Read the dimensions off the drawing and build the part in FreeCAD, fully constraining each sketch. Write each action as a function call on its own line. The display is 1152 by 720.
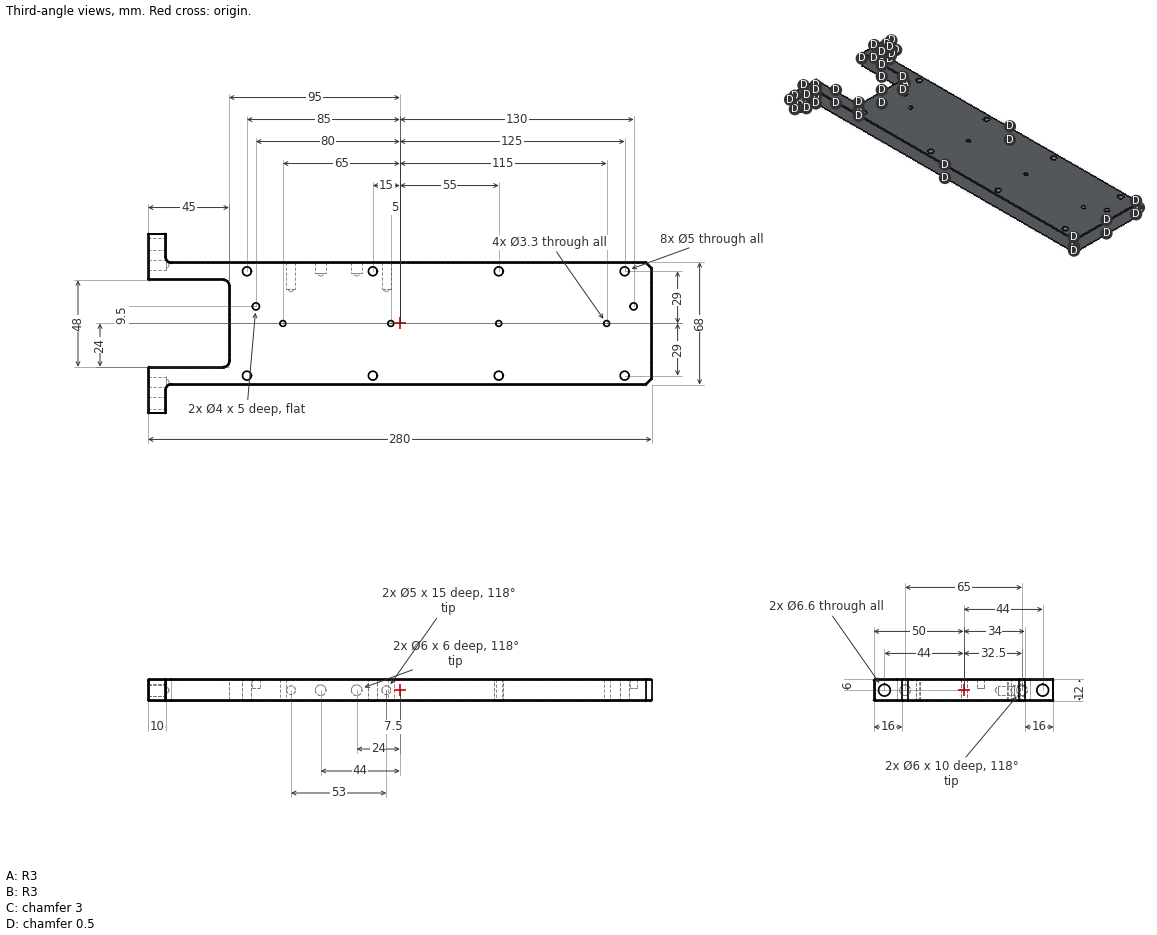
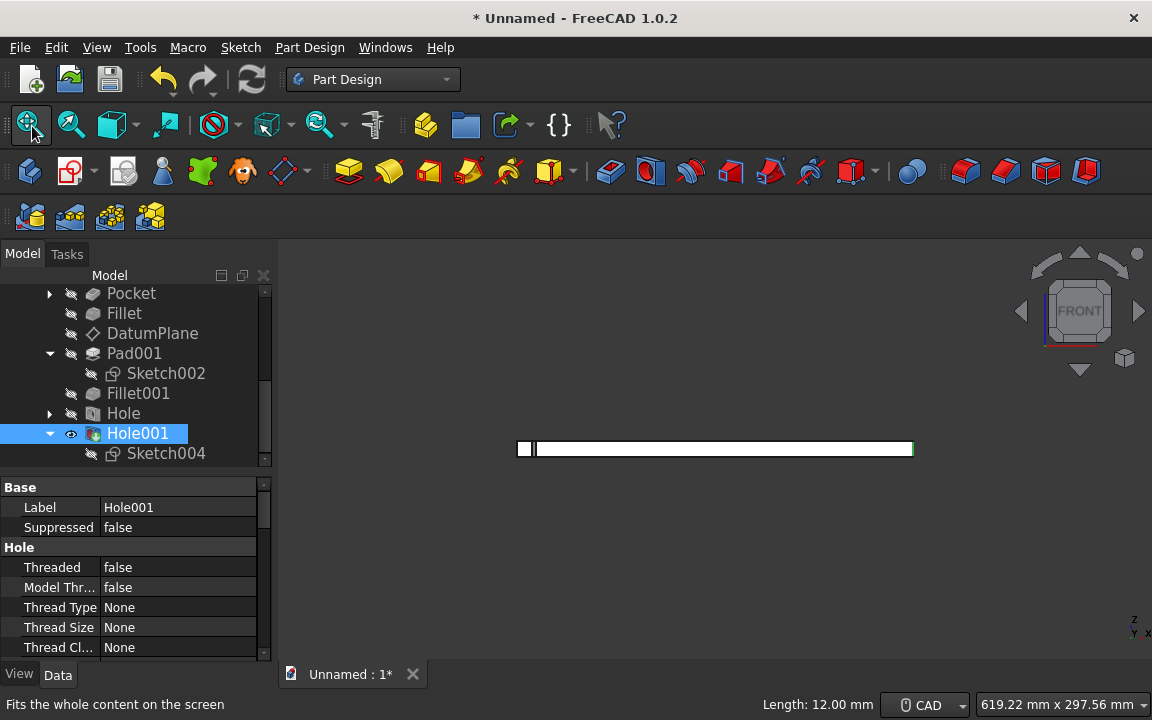
key(3)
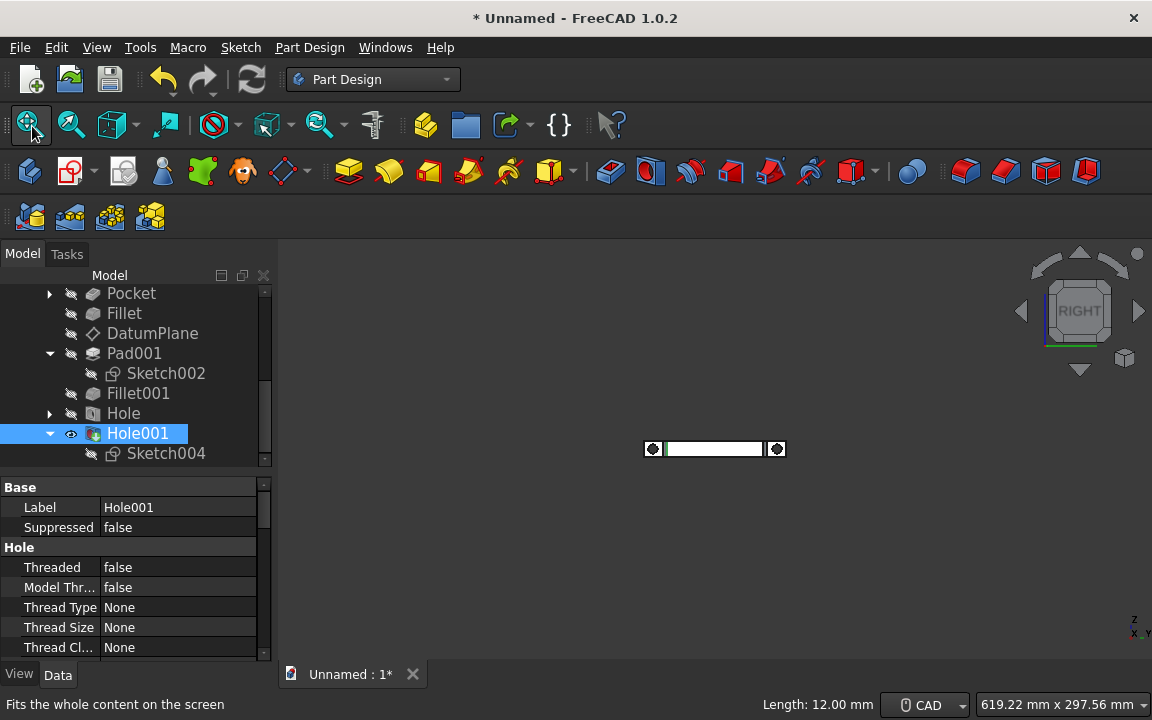
click(32, 126)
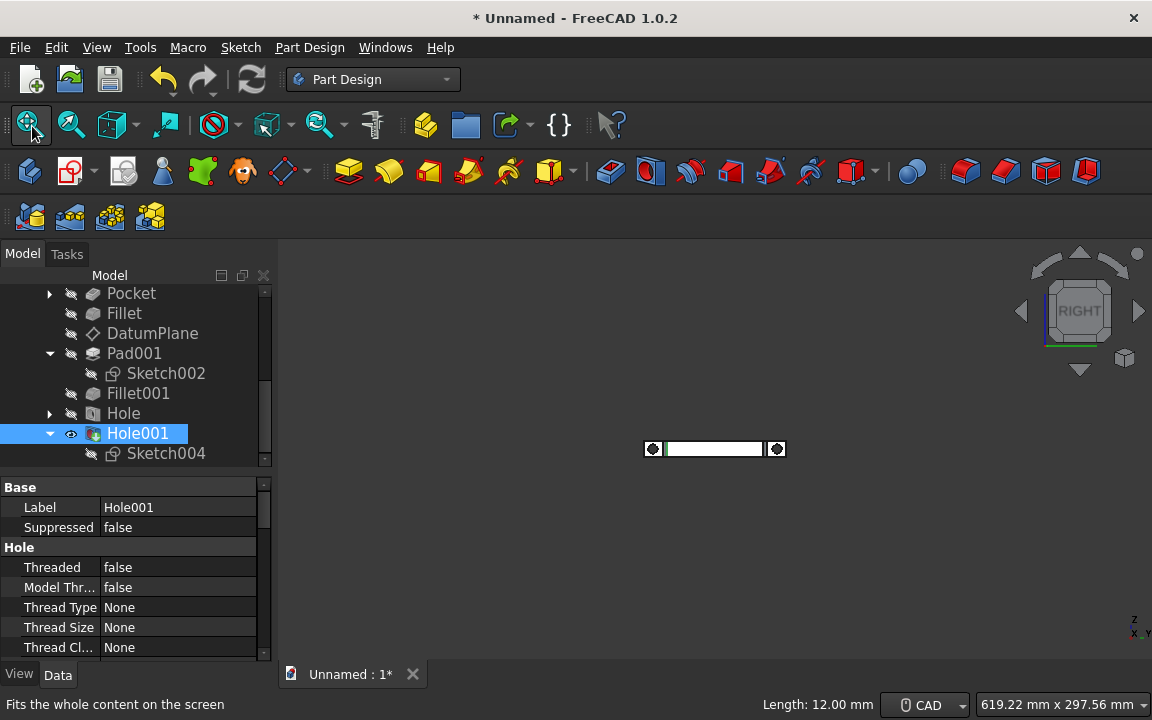
click(763, 448, ctrl)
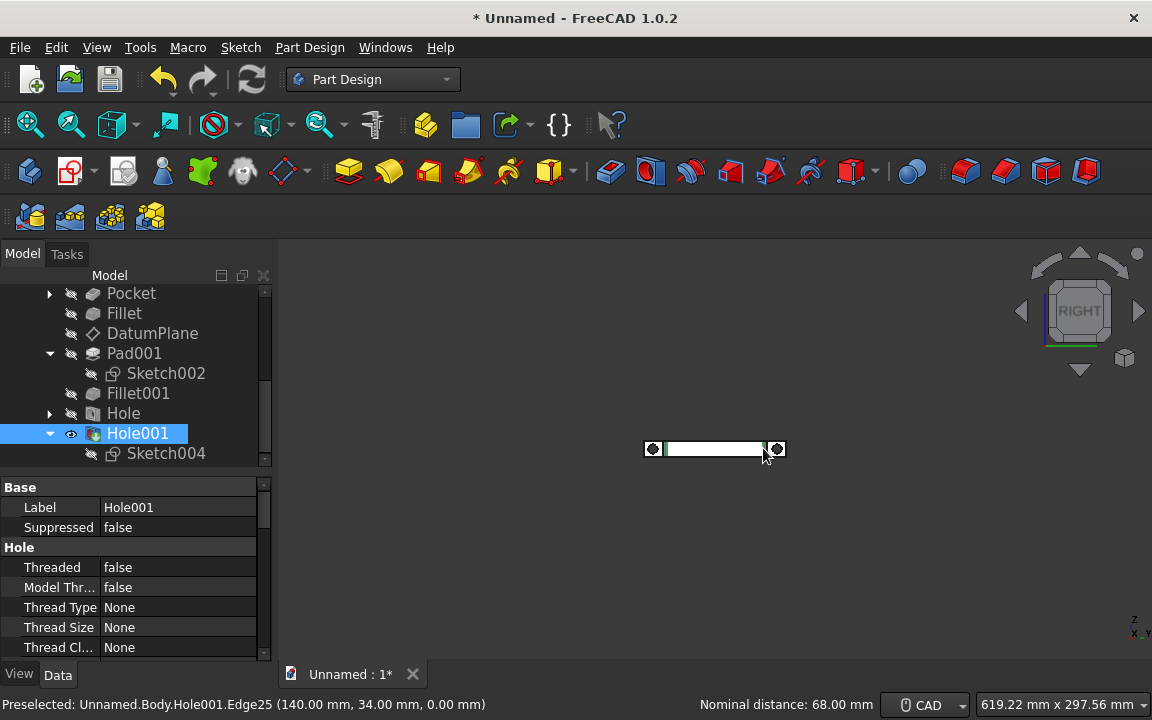
click(1006, 172)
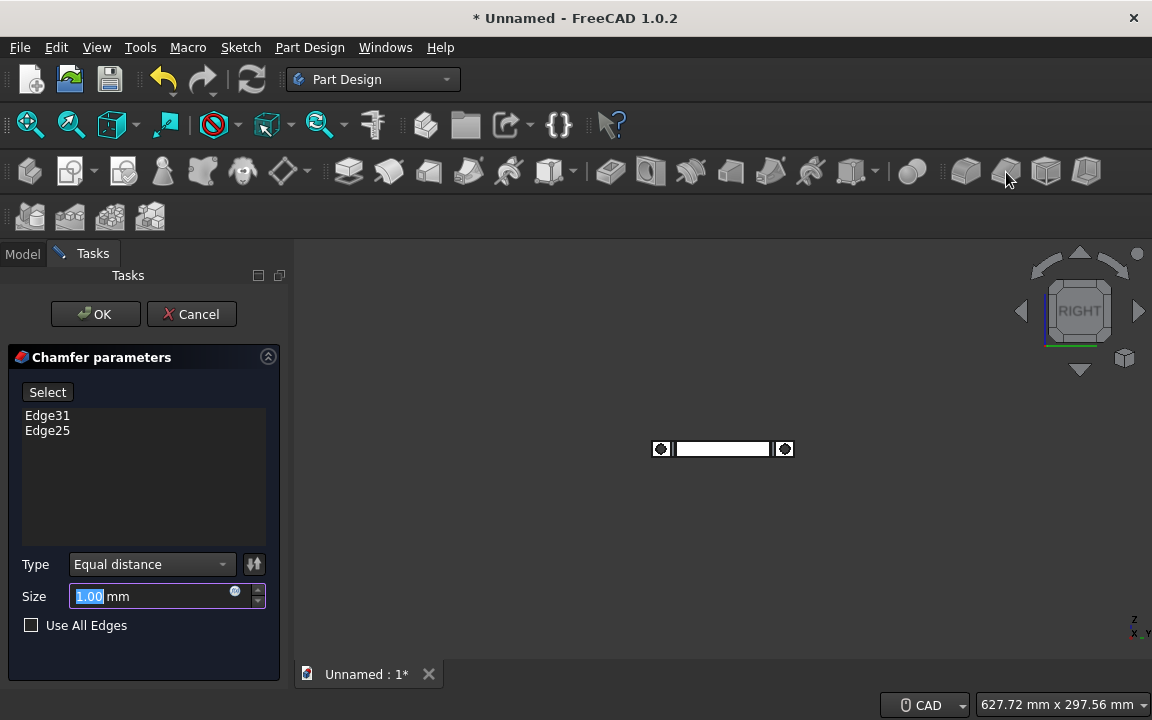
text(3)
key(Tab)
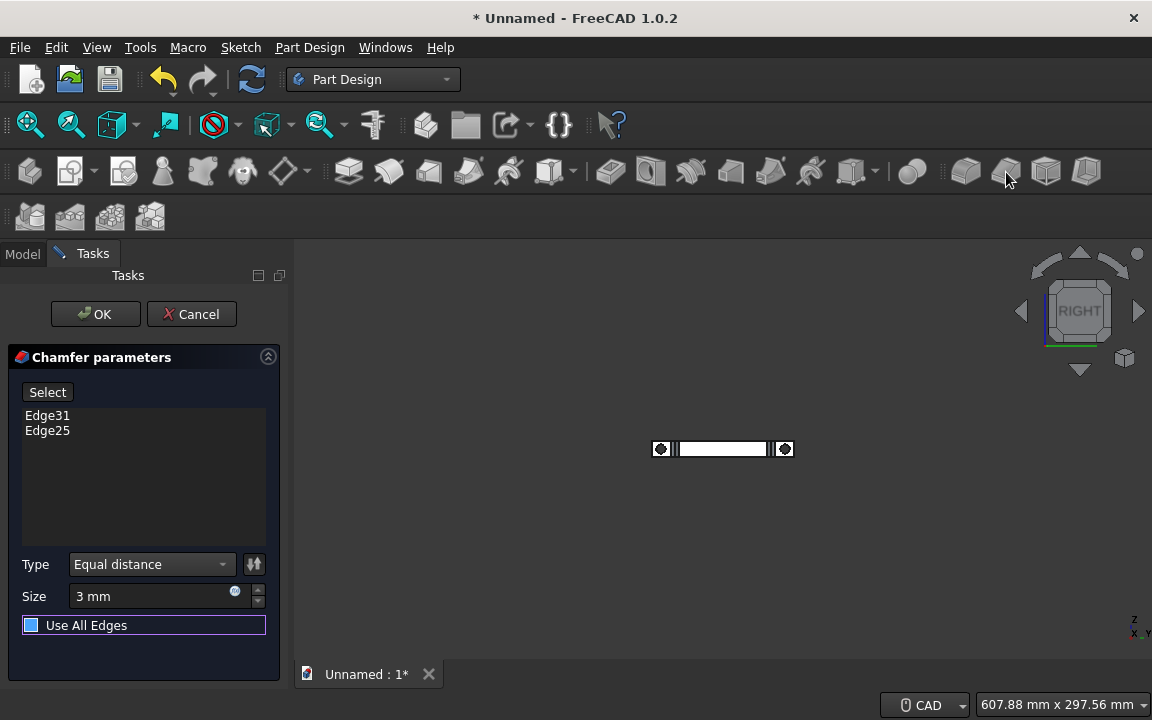
click(96, 314)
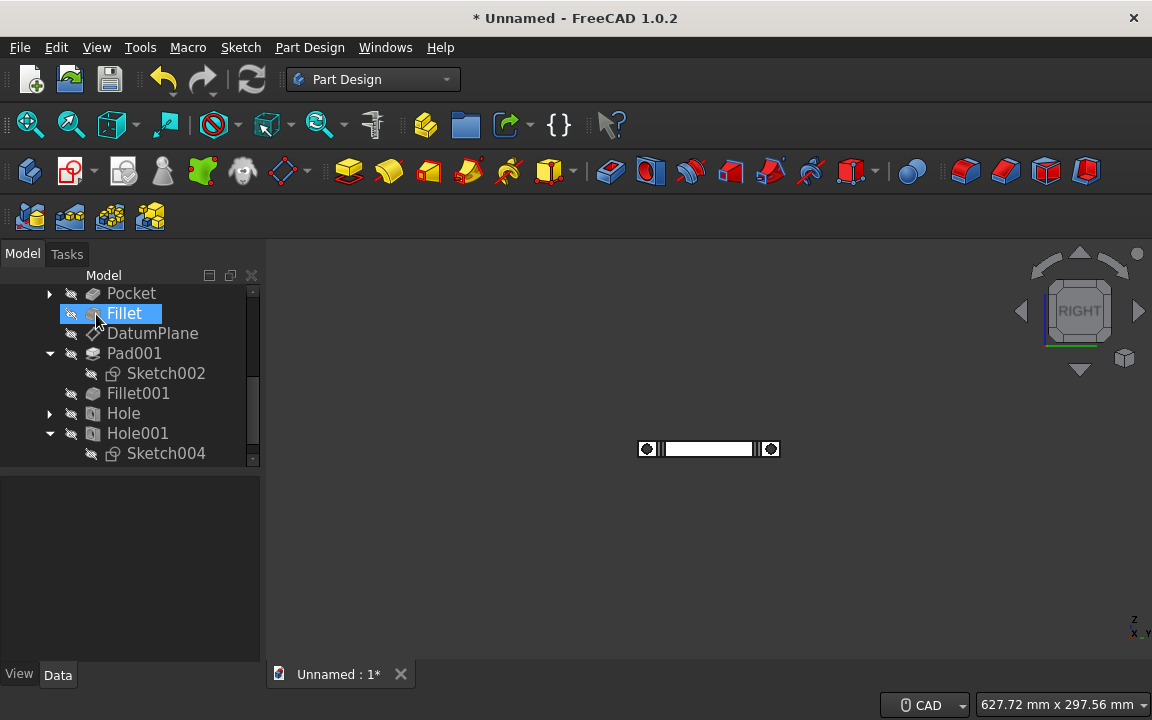
key(v)
key(f)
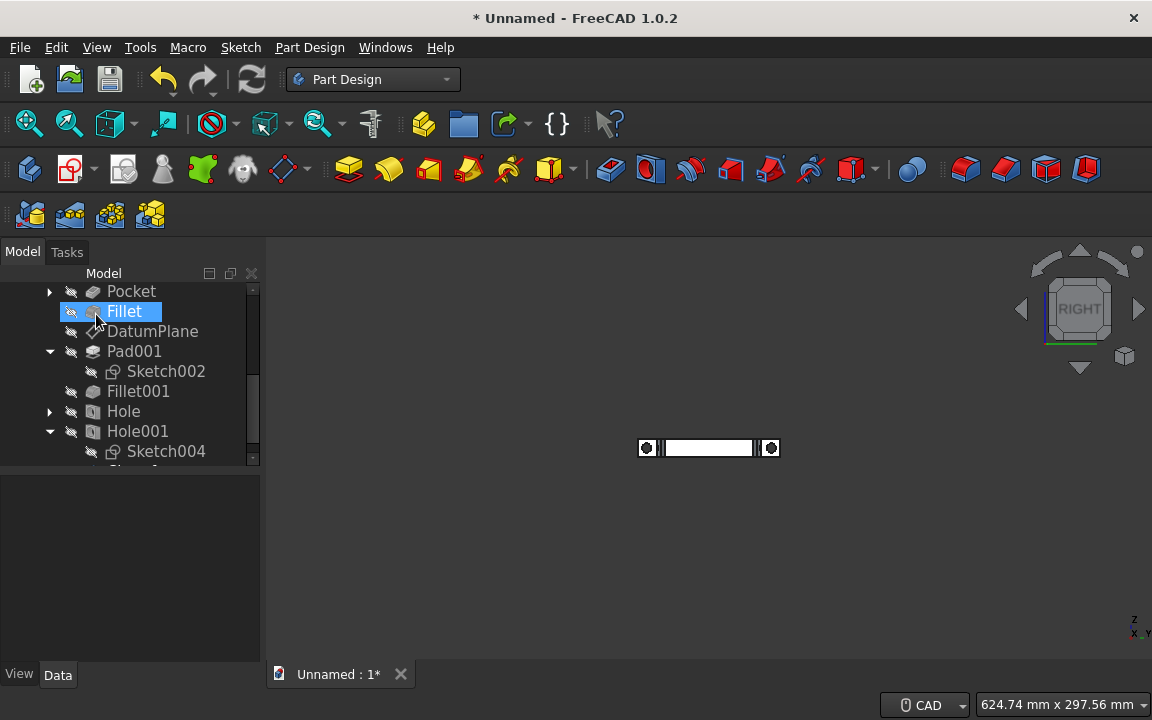
click(638, 447)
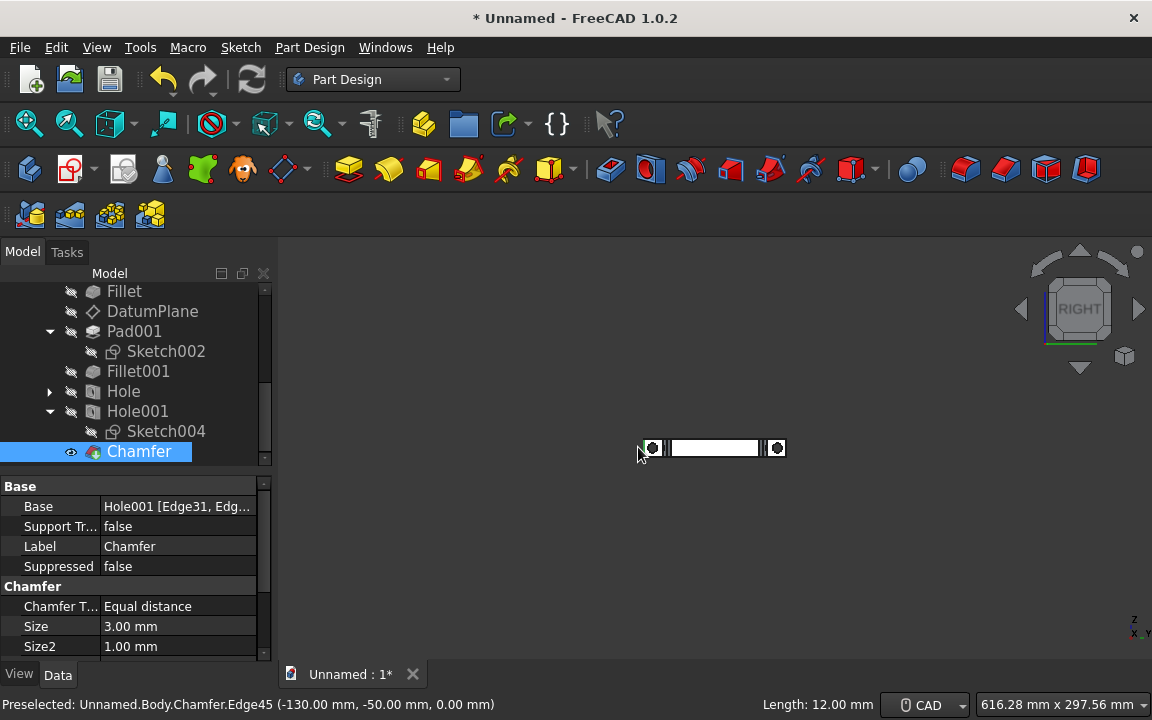
click(786, 447, ctrl)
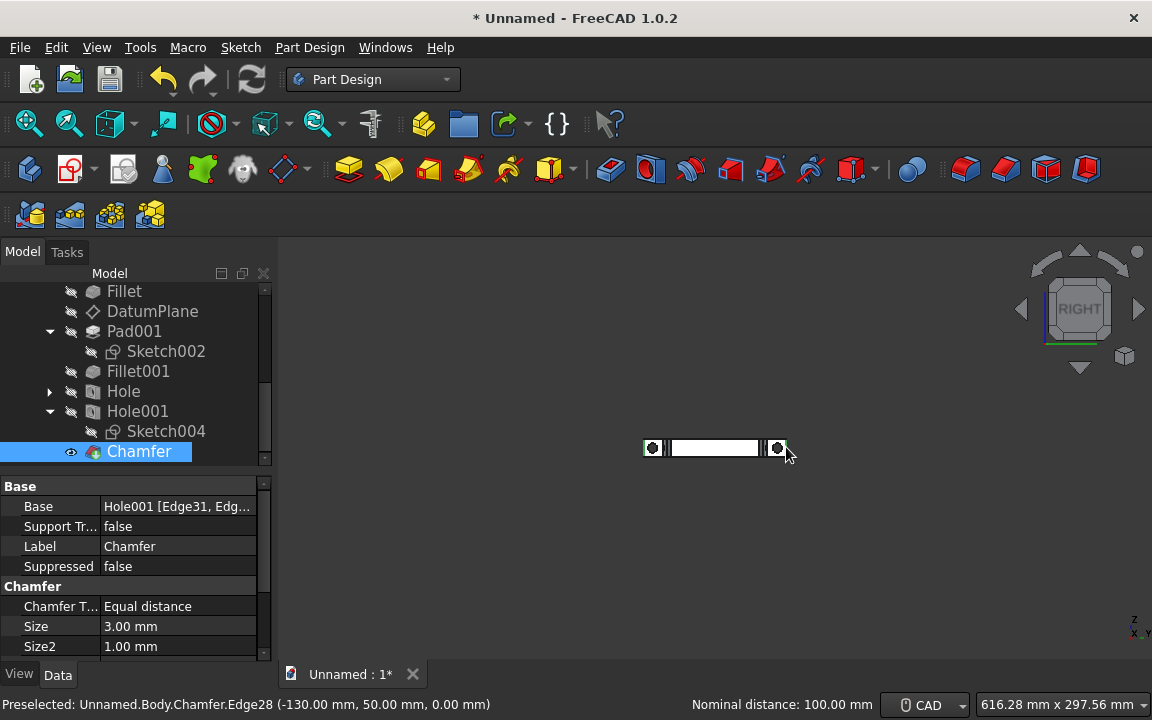
key(0)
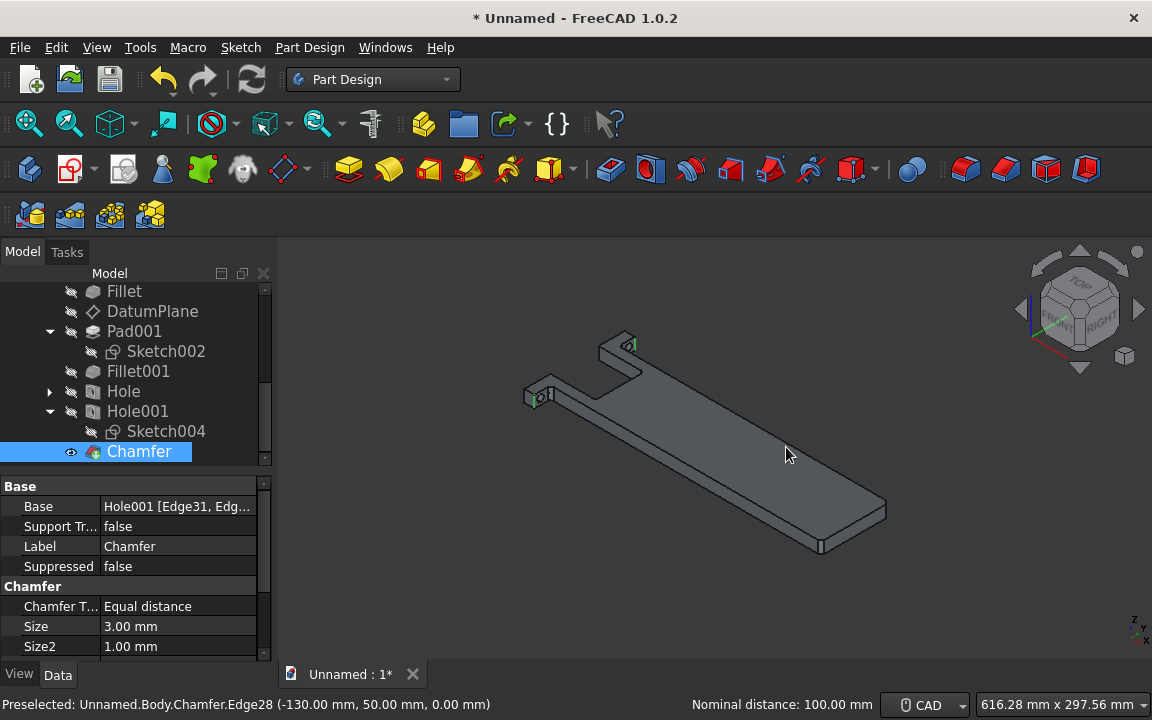
click(795, 486, ctrl)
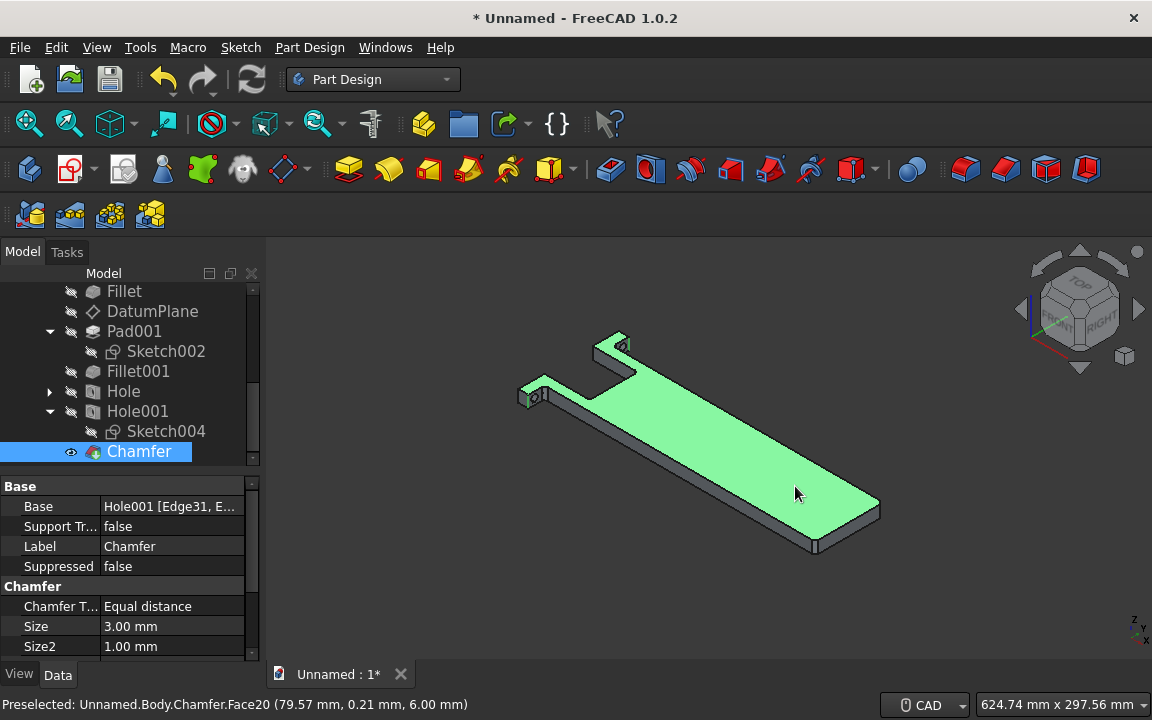
key(2)